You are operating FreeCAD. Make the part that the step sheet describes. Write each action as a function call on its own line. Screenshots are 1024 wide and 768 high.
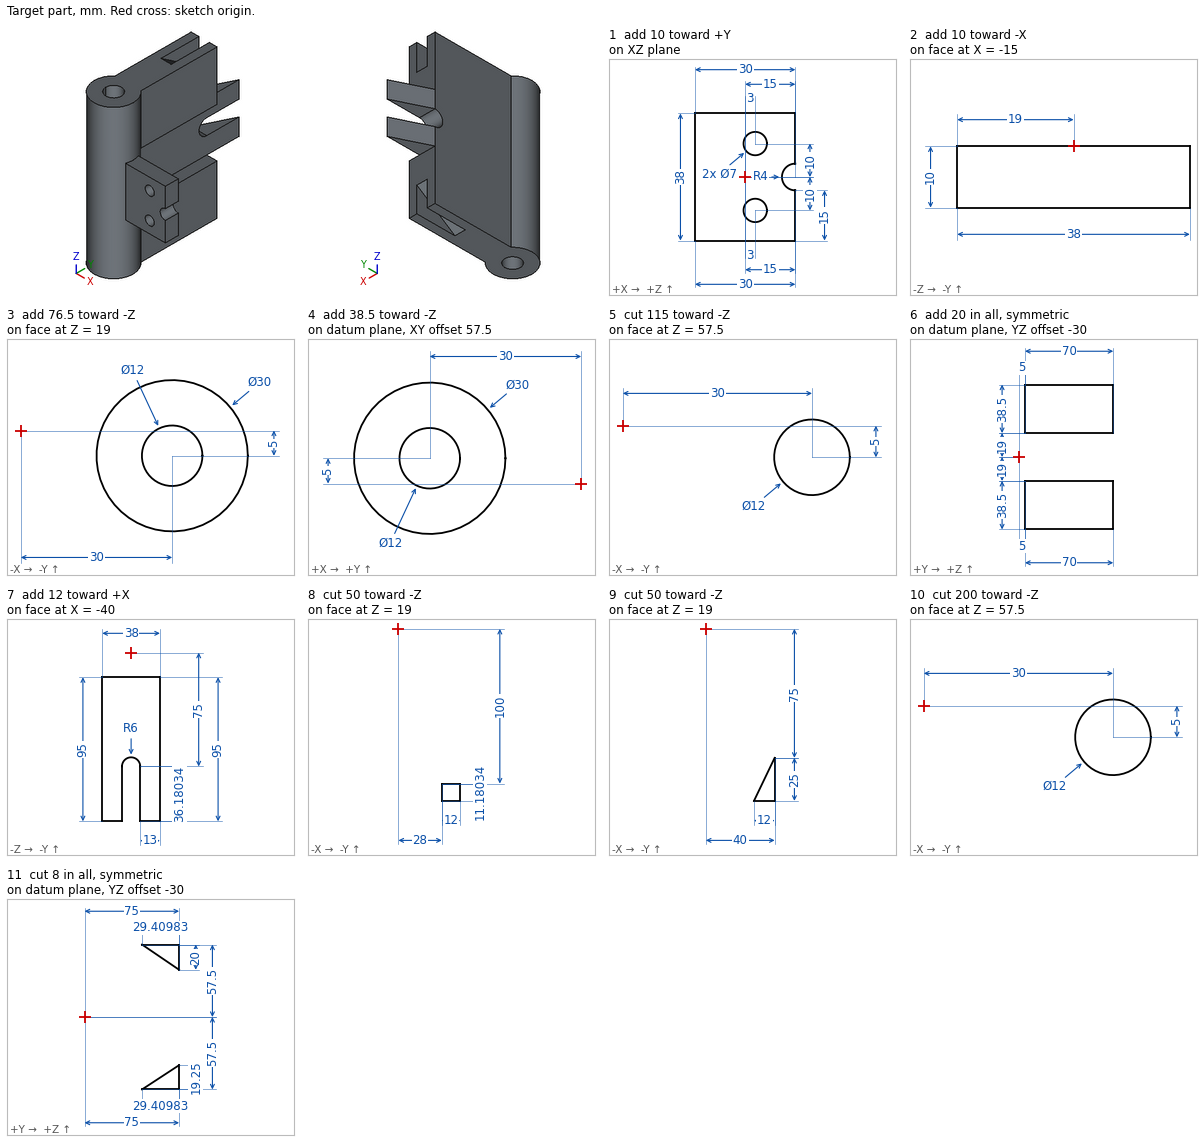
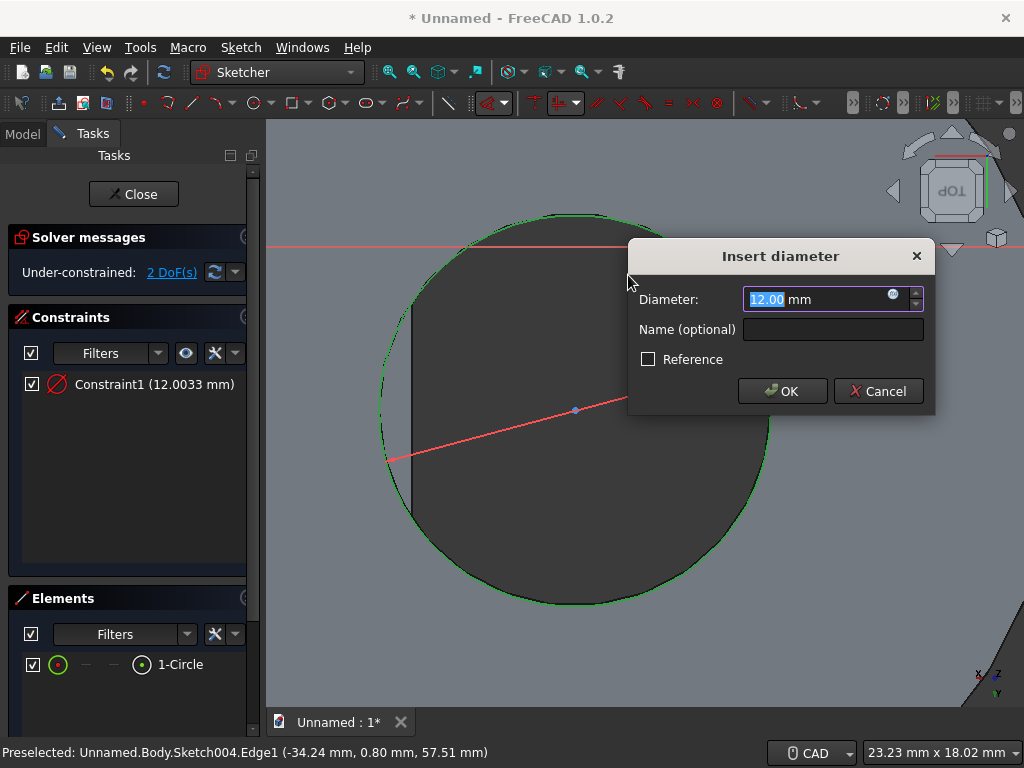
text(12)
key(Return)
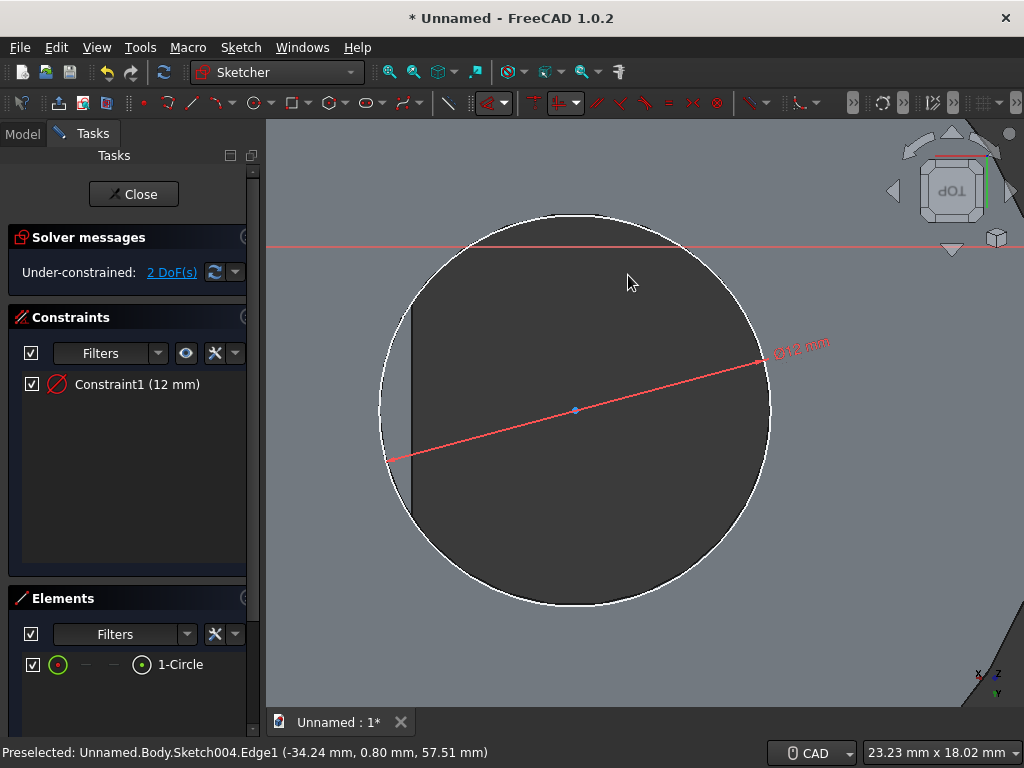
click(575, 411)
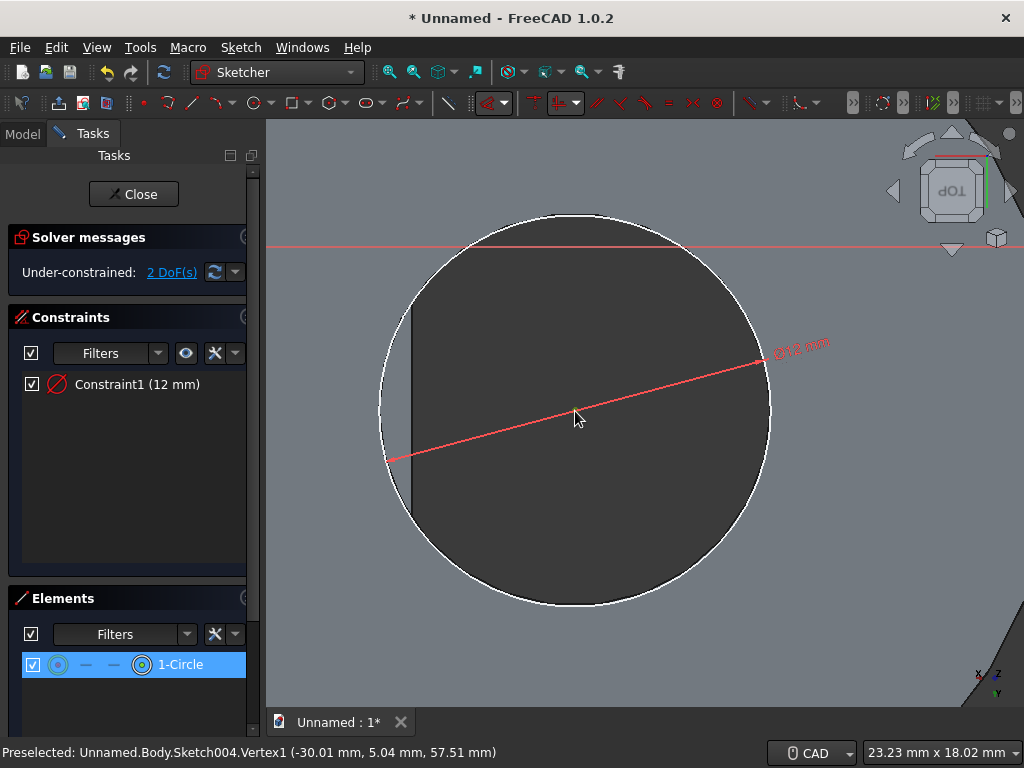
click(506, 104)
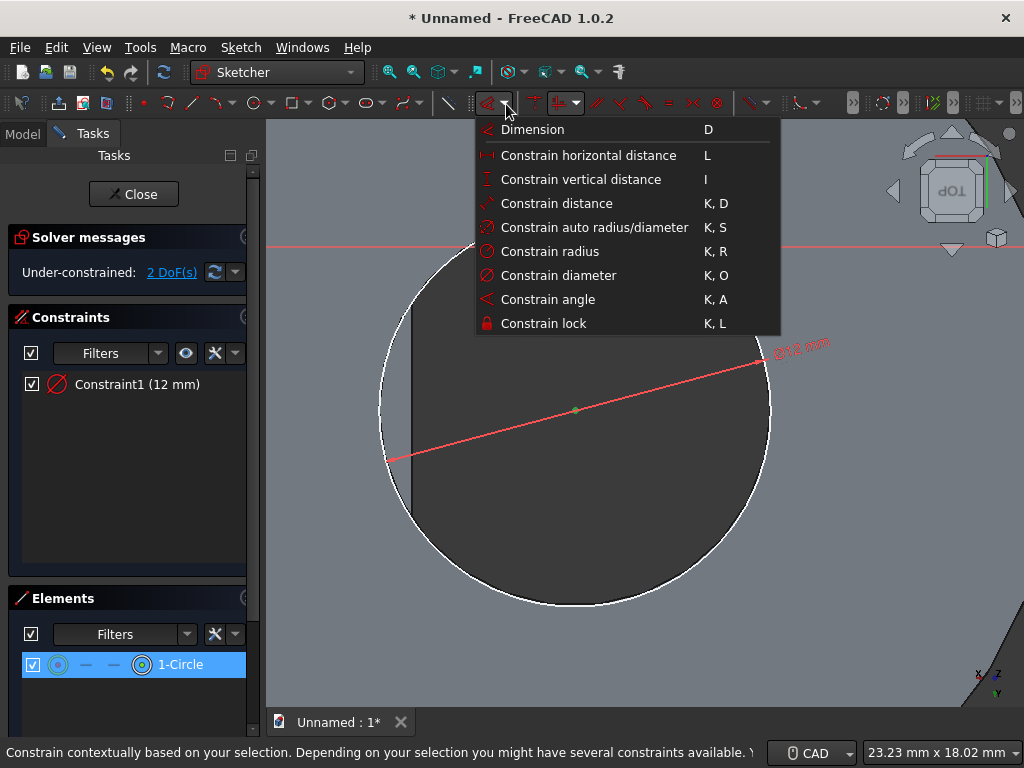
click(628, 179)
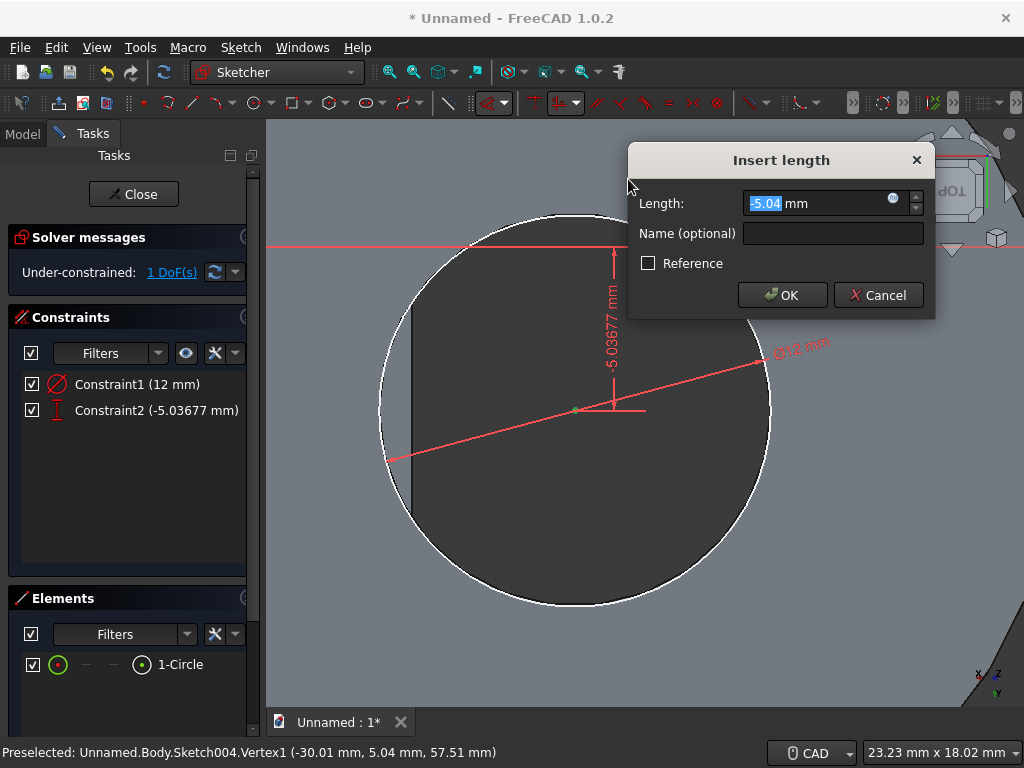
text(-5)
key(Return)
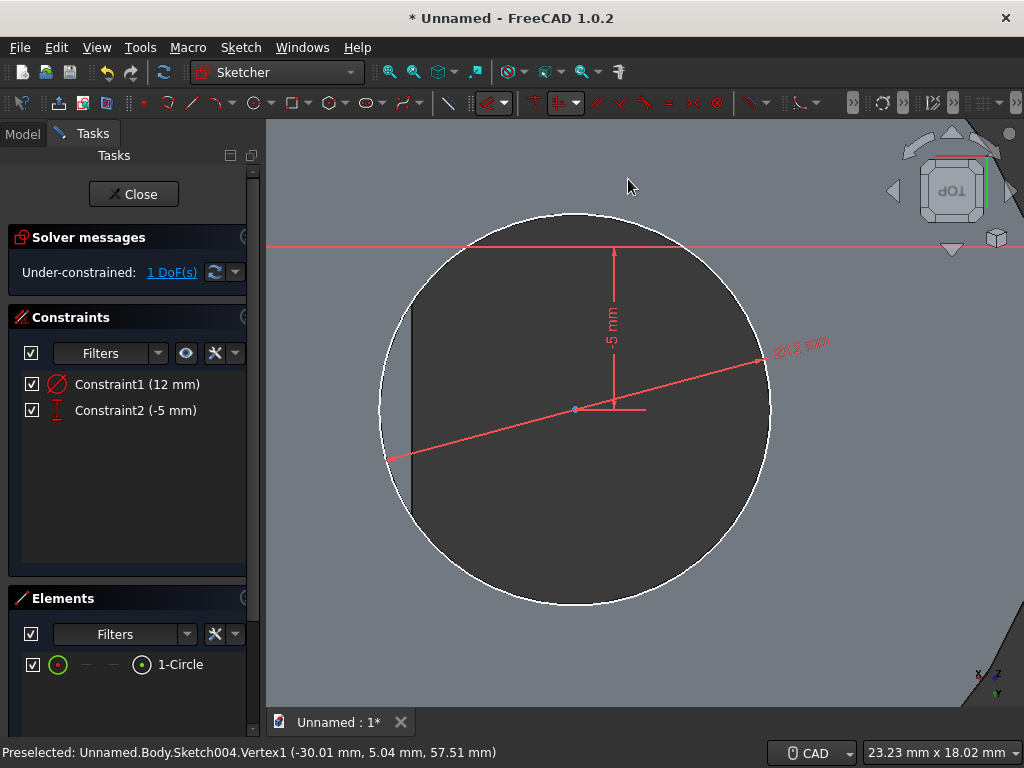
click(575, 410)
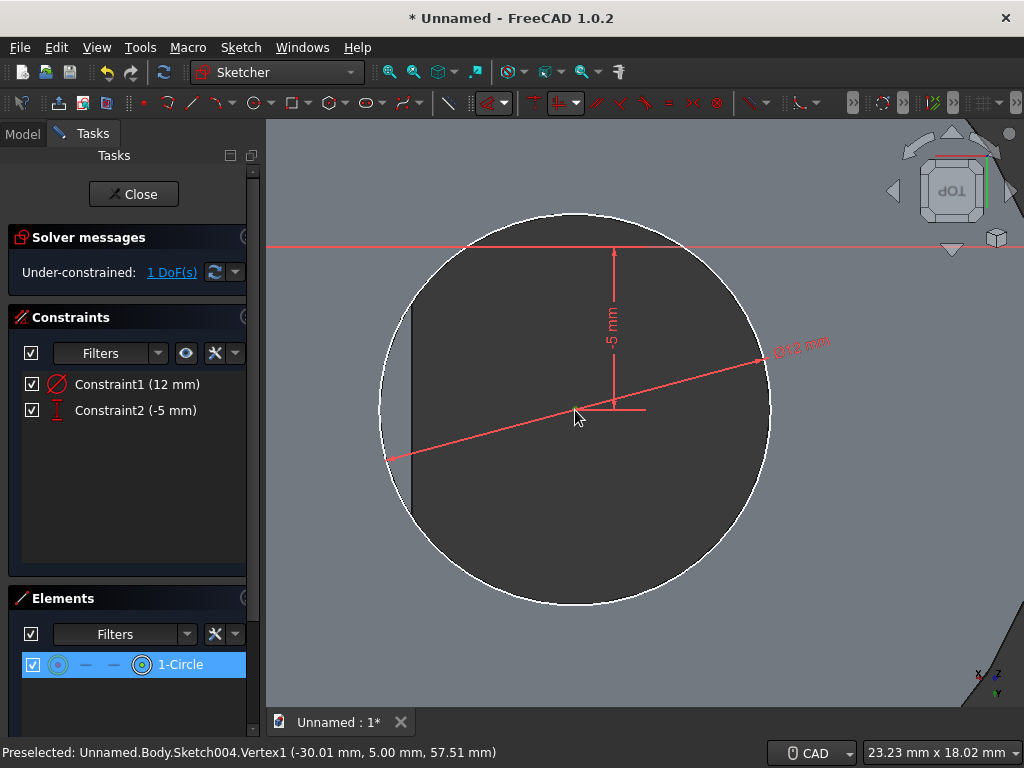
key(l)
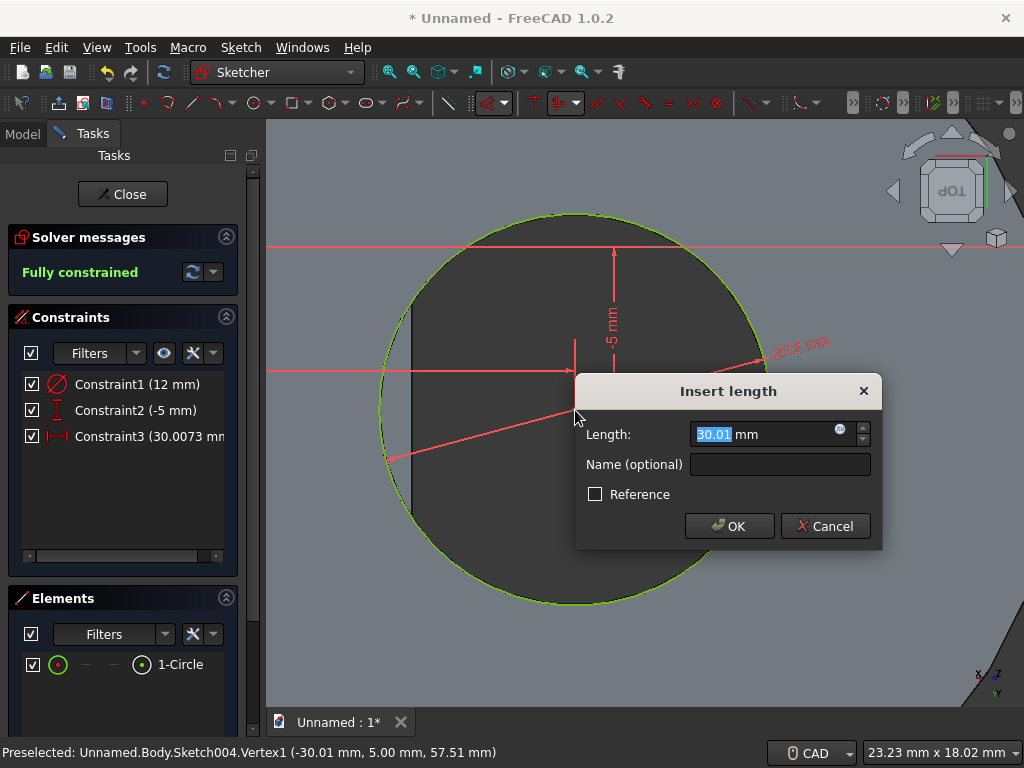
text(30)
key(Return)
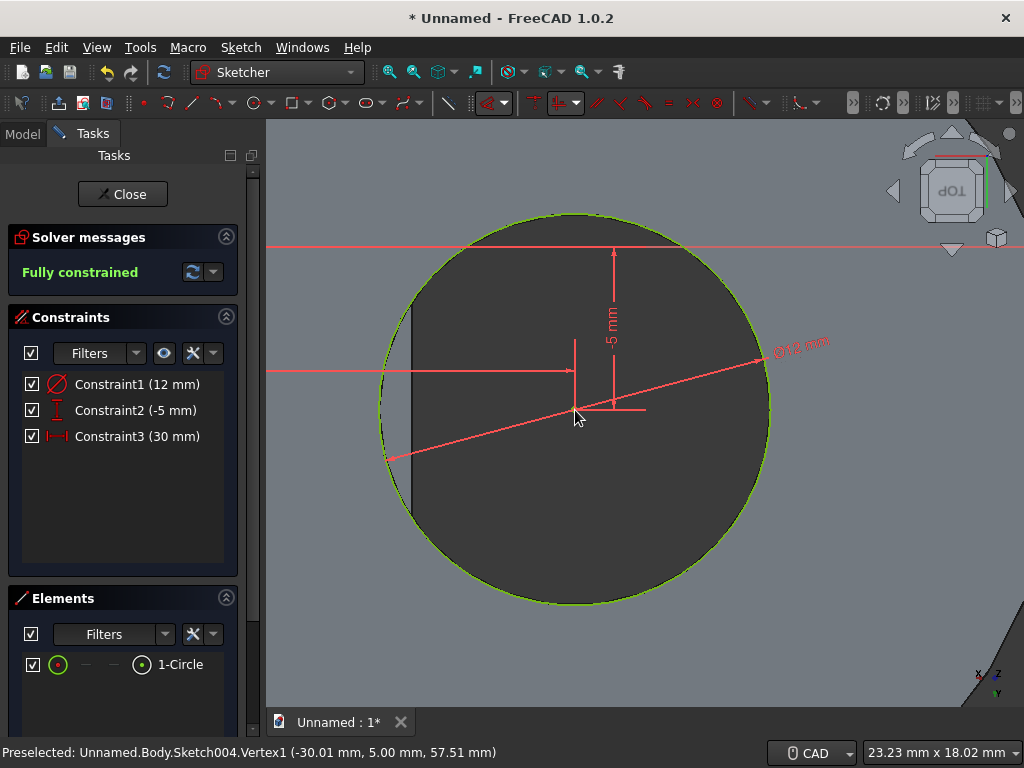
click(123, 194)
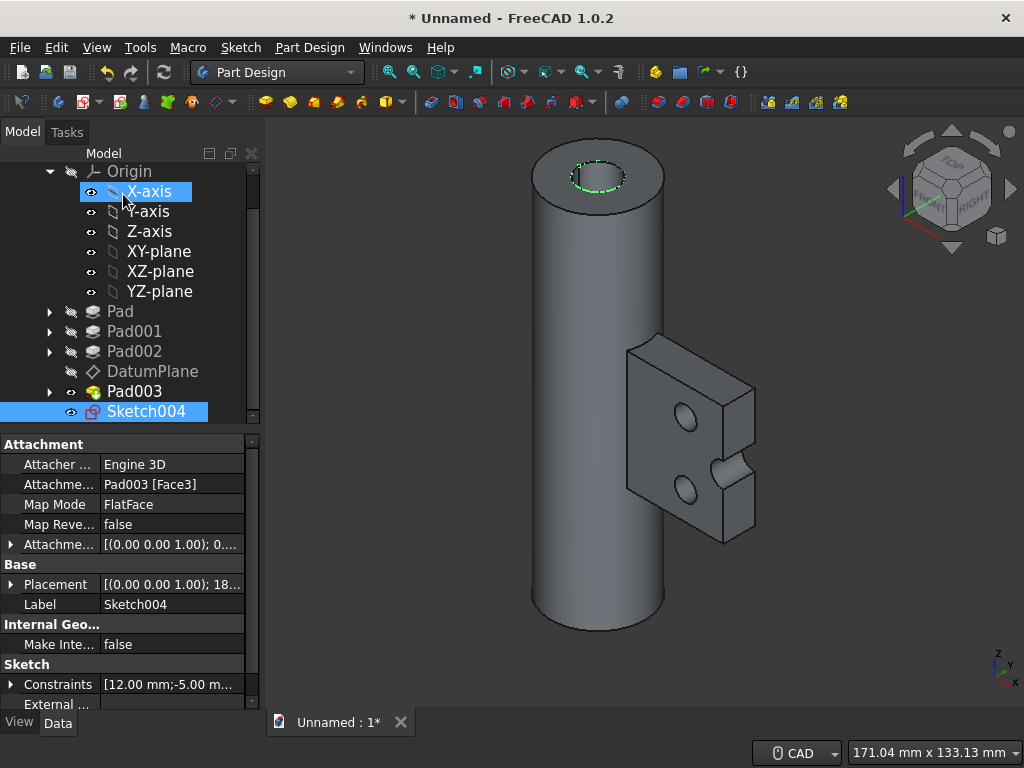
click(432, 102)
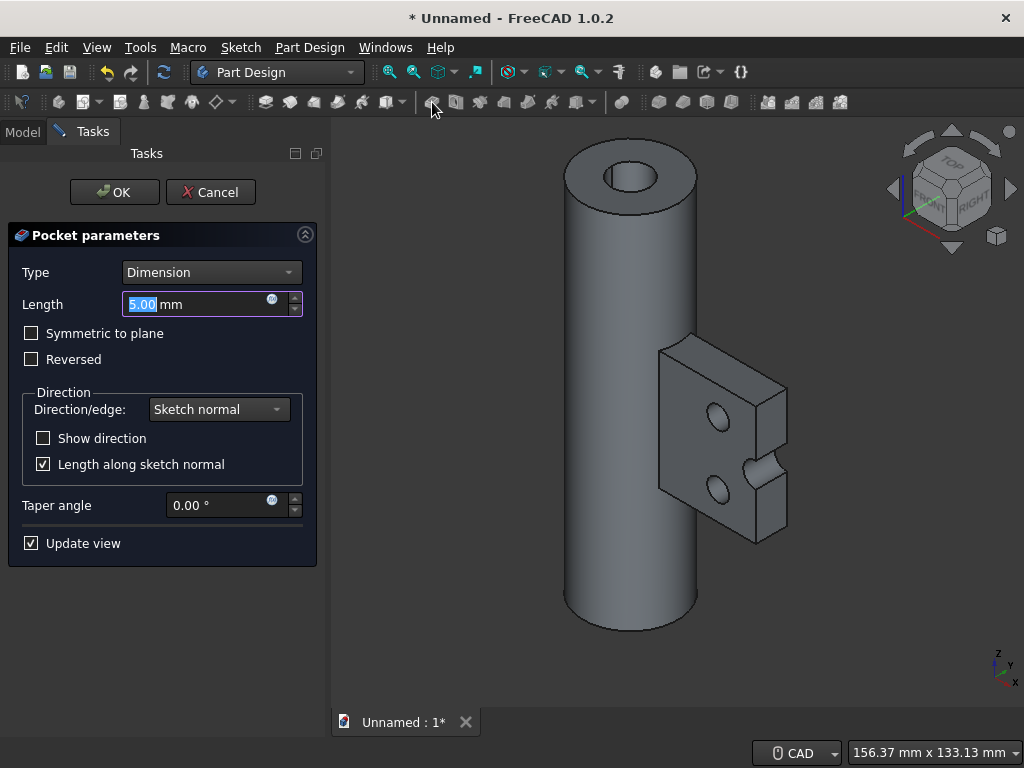
text(115)
key(Tab)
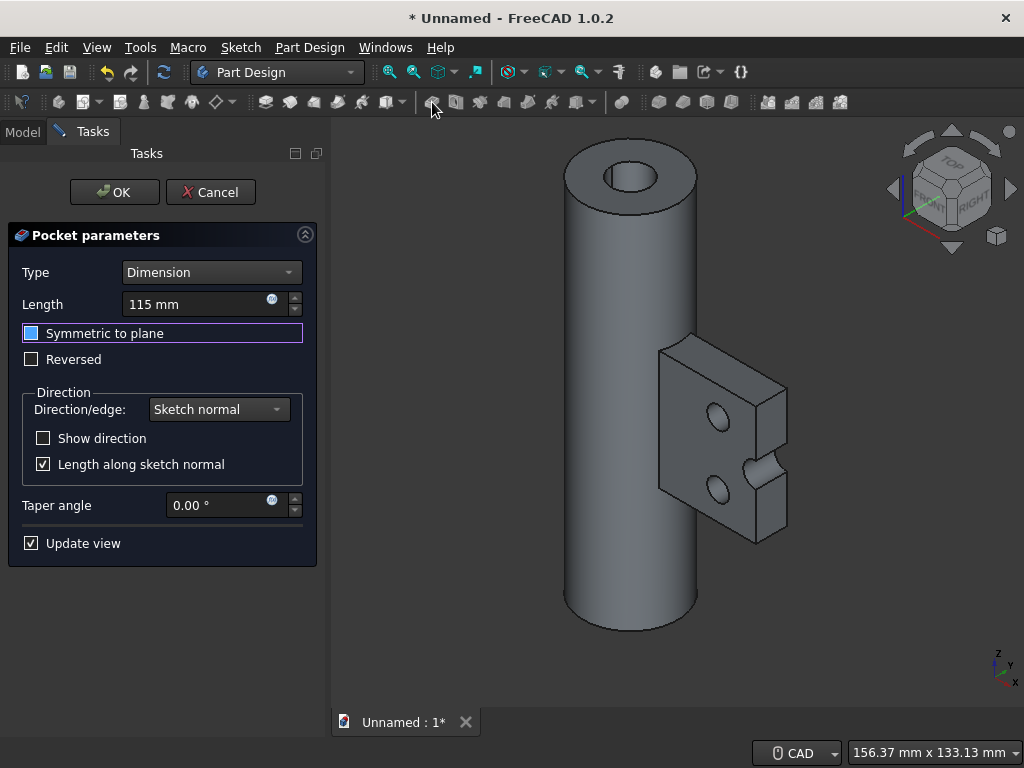
click(115, 192)